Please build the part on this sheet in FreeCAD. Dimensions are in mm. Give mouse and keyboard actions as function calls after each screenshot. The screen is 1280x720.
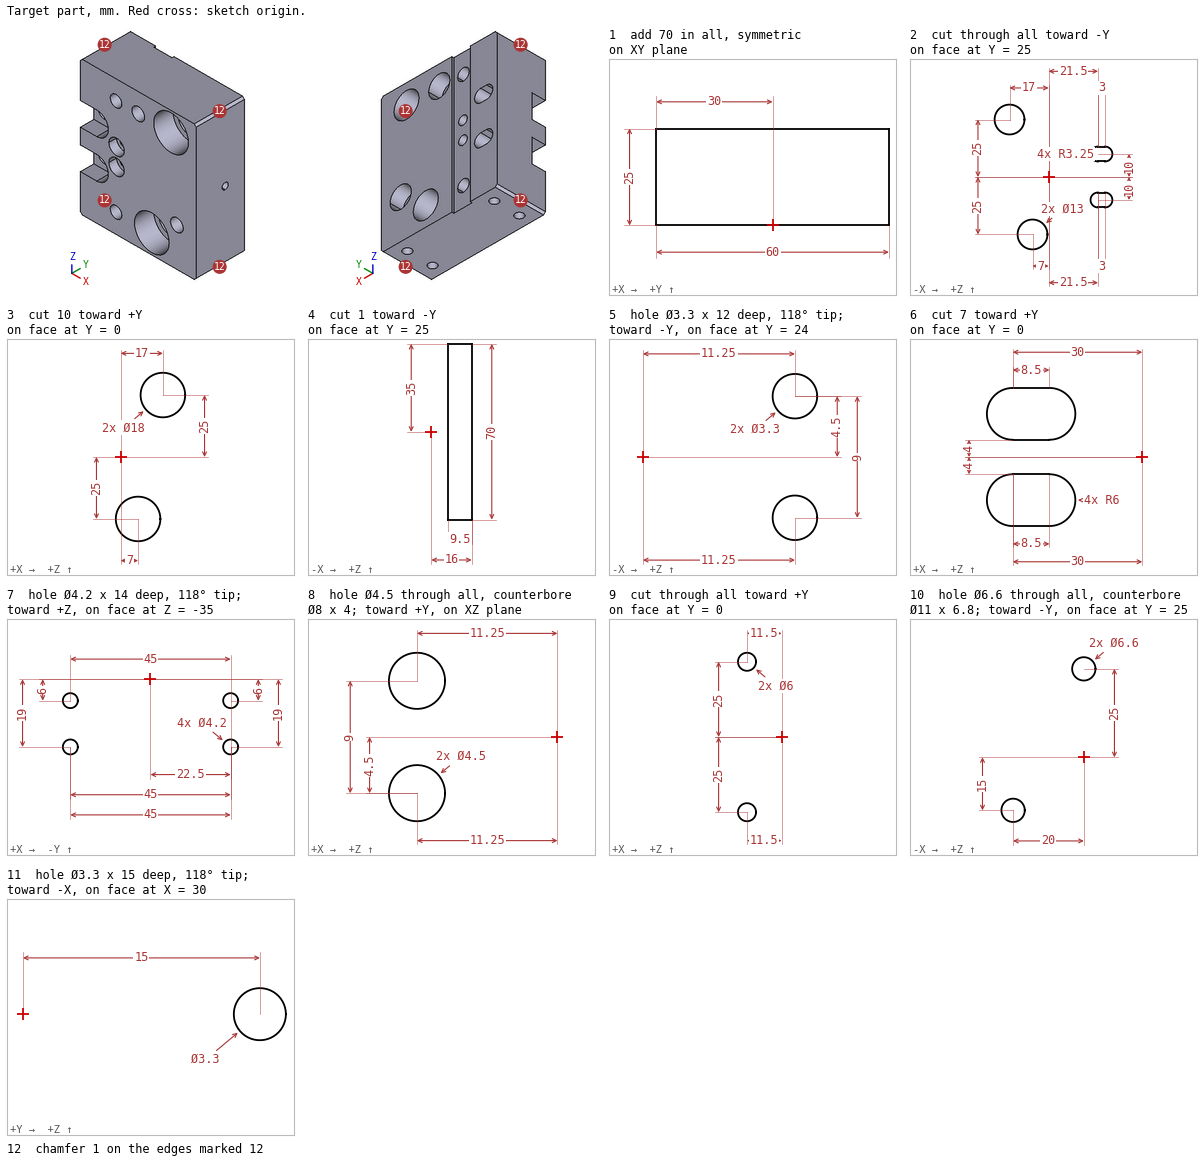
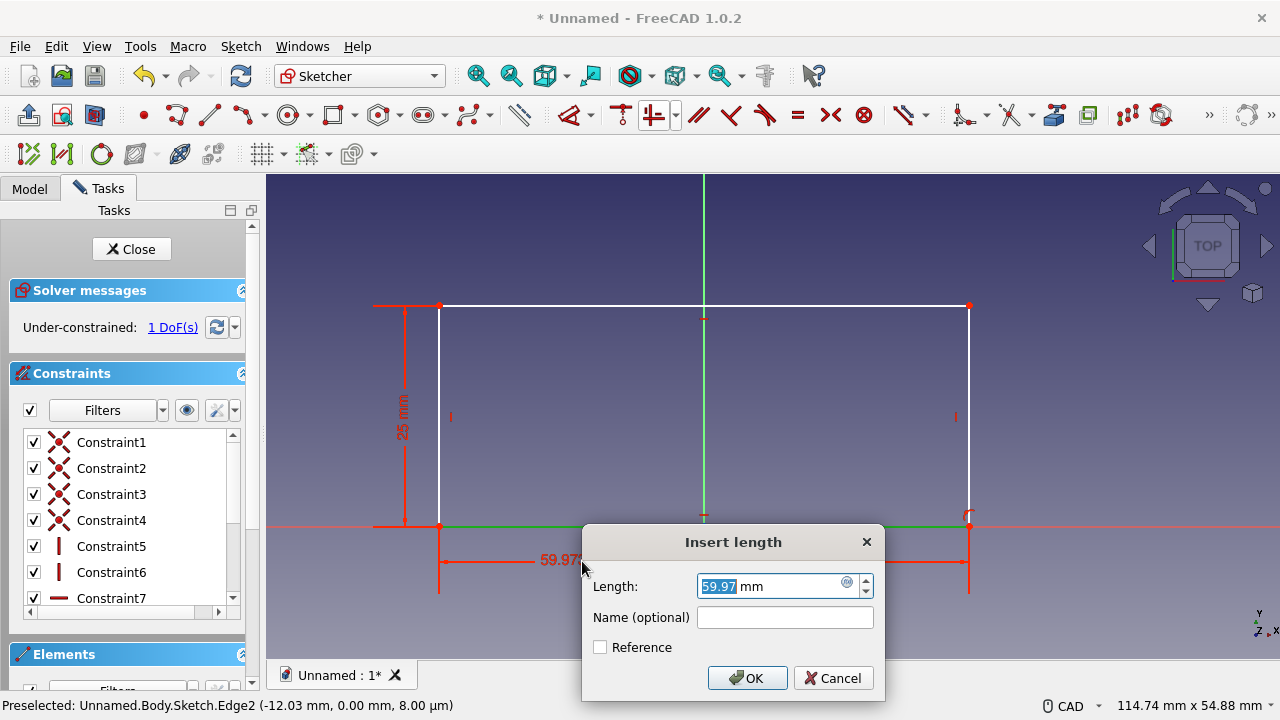
text(60)
key(Return)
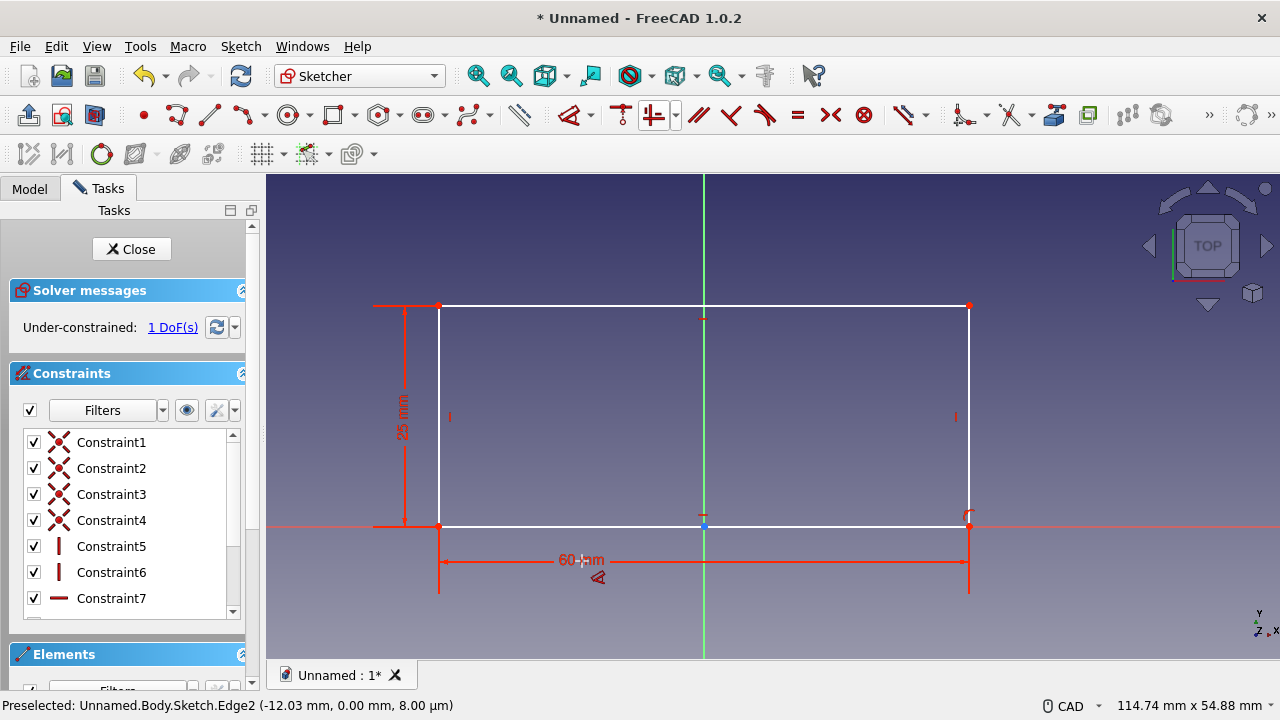
click(439, 306)
click(510, 561)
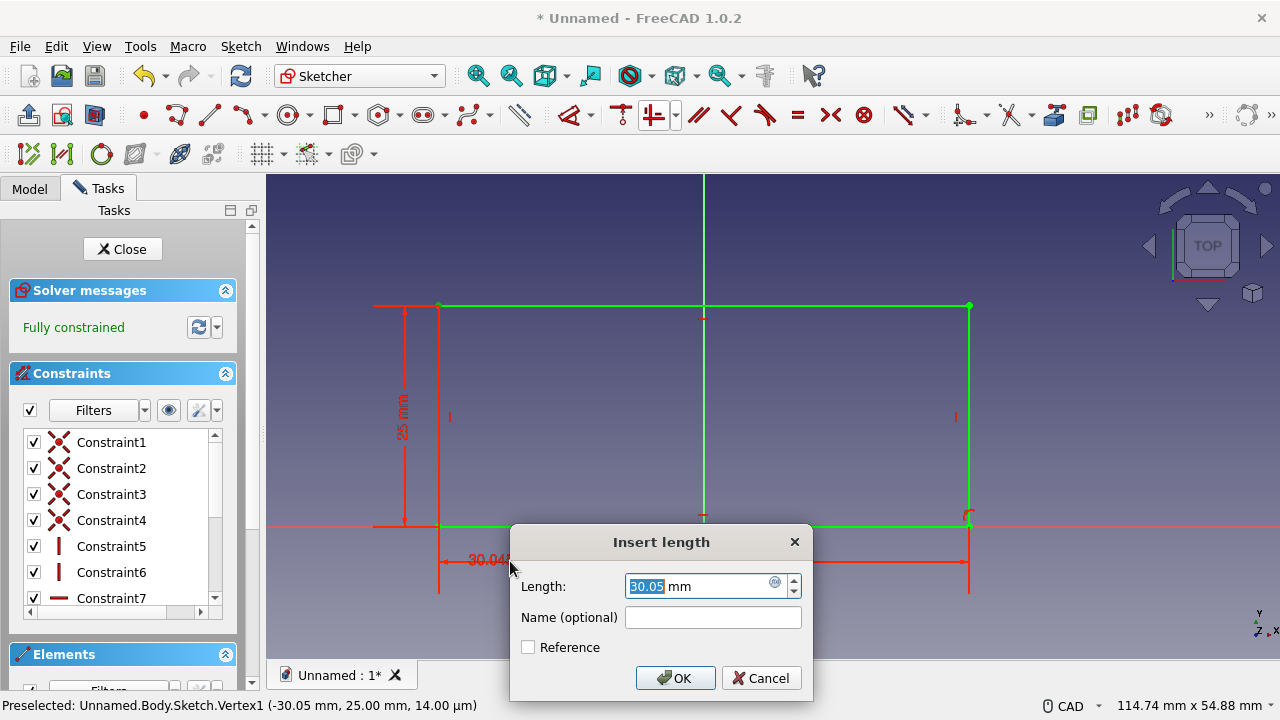
text(30)
key(Return)
key(Escape)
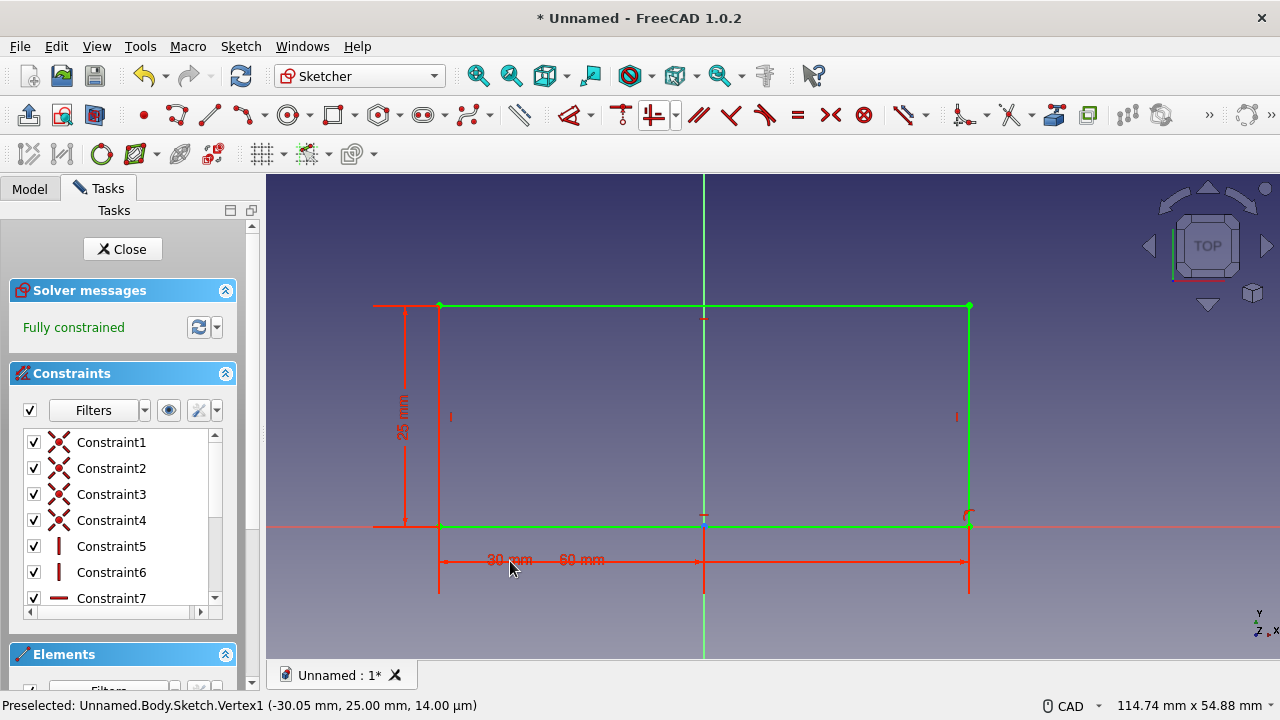
click(123, 249)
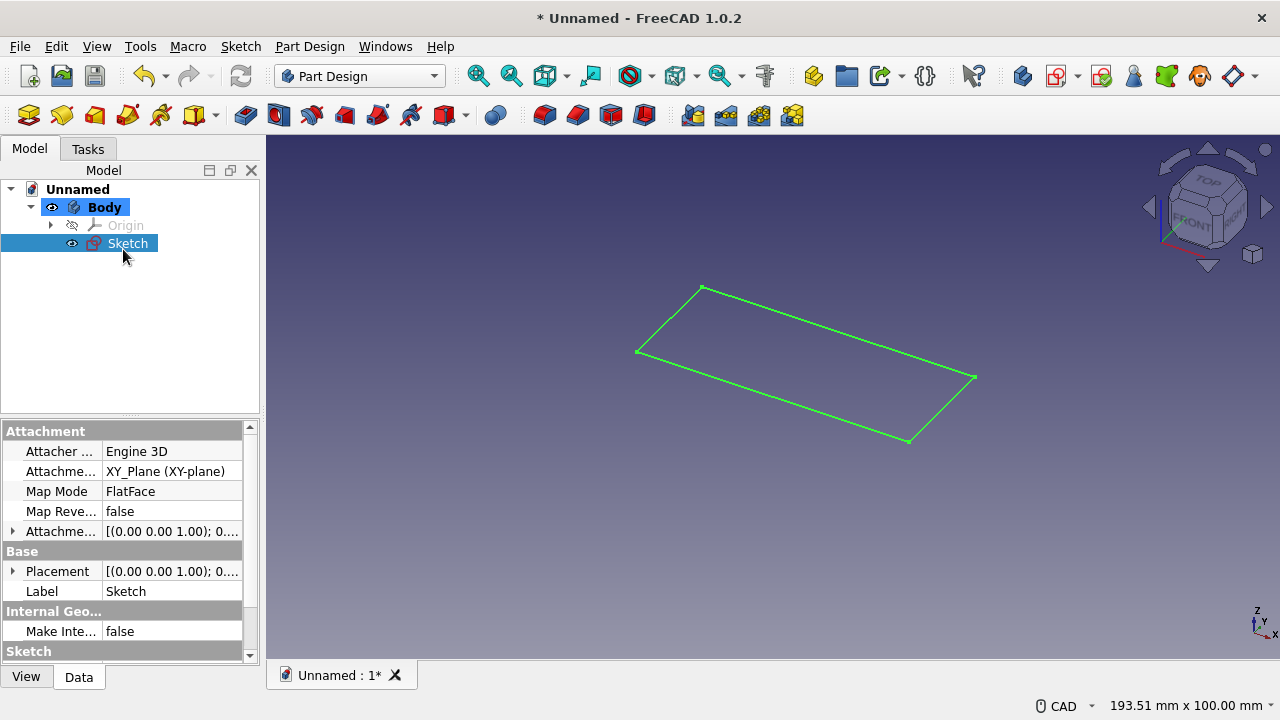
click(29, 116)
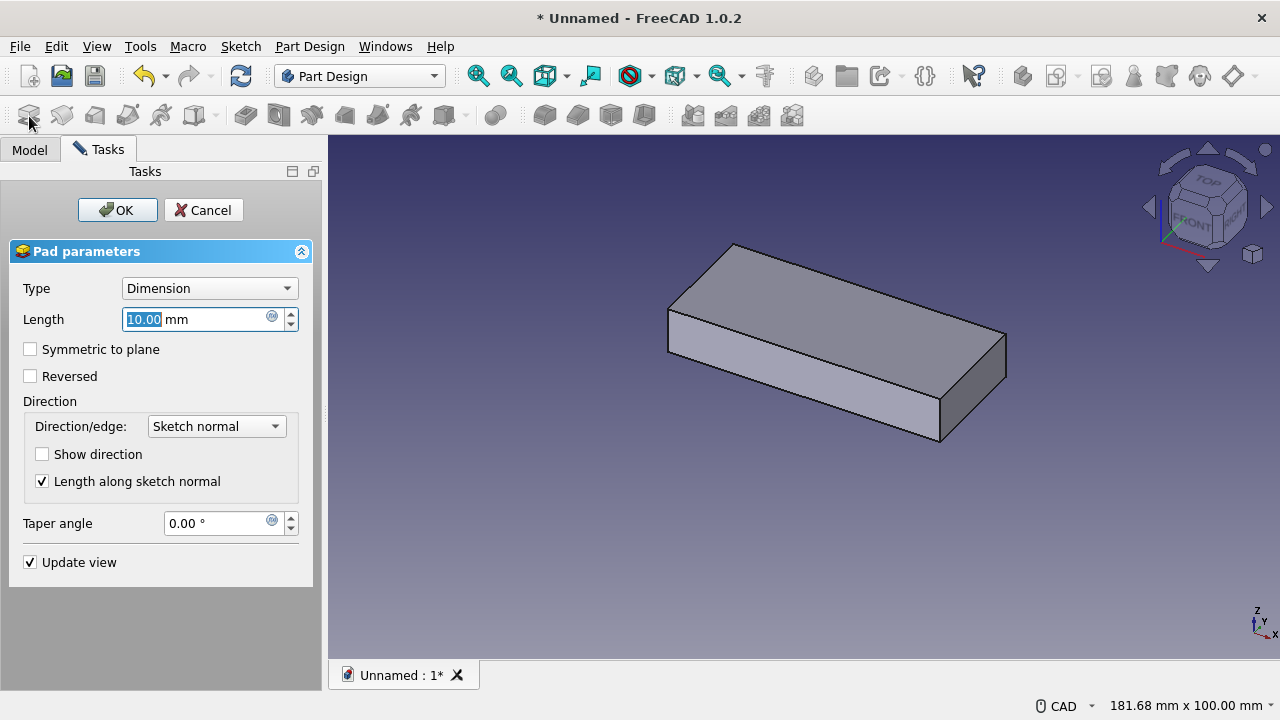
text(70)
key(Tab)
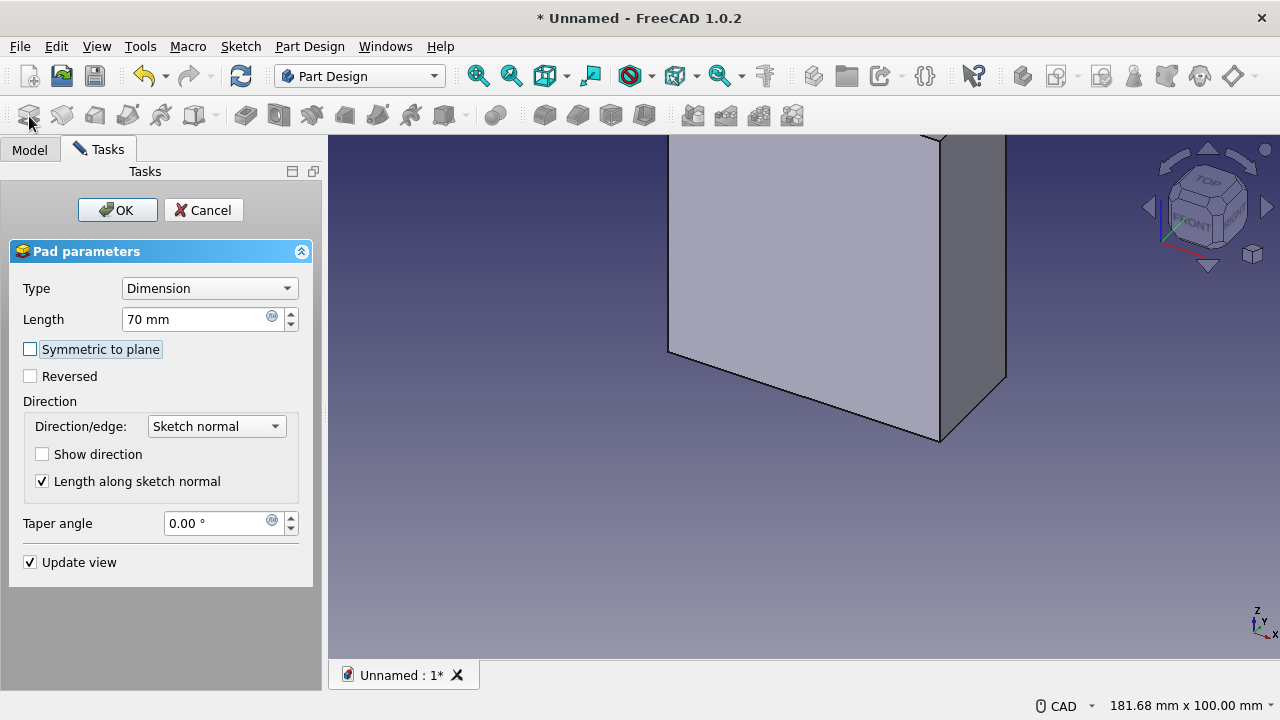
click(31, 349)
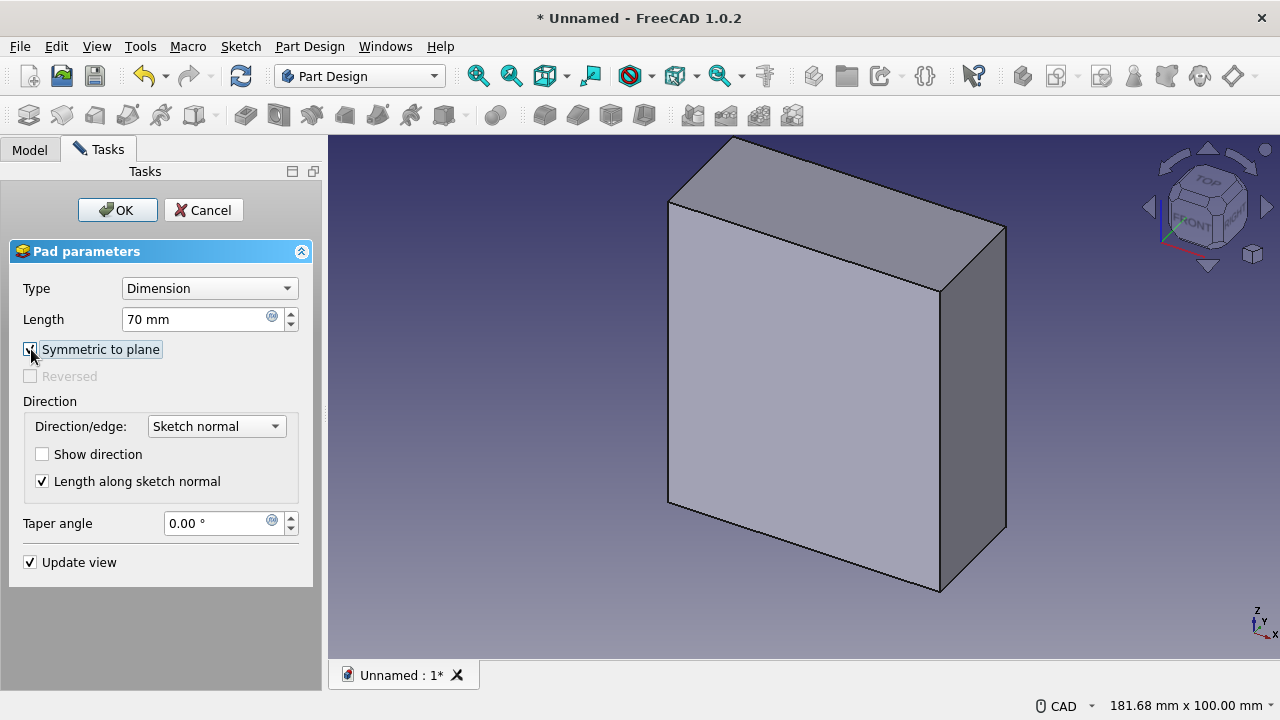
click(118, 210)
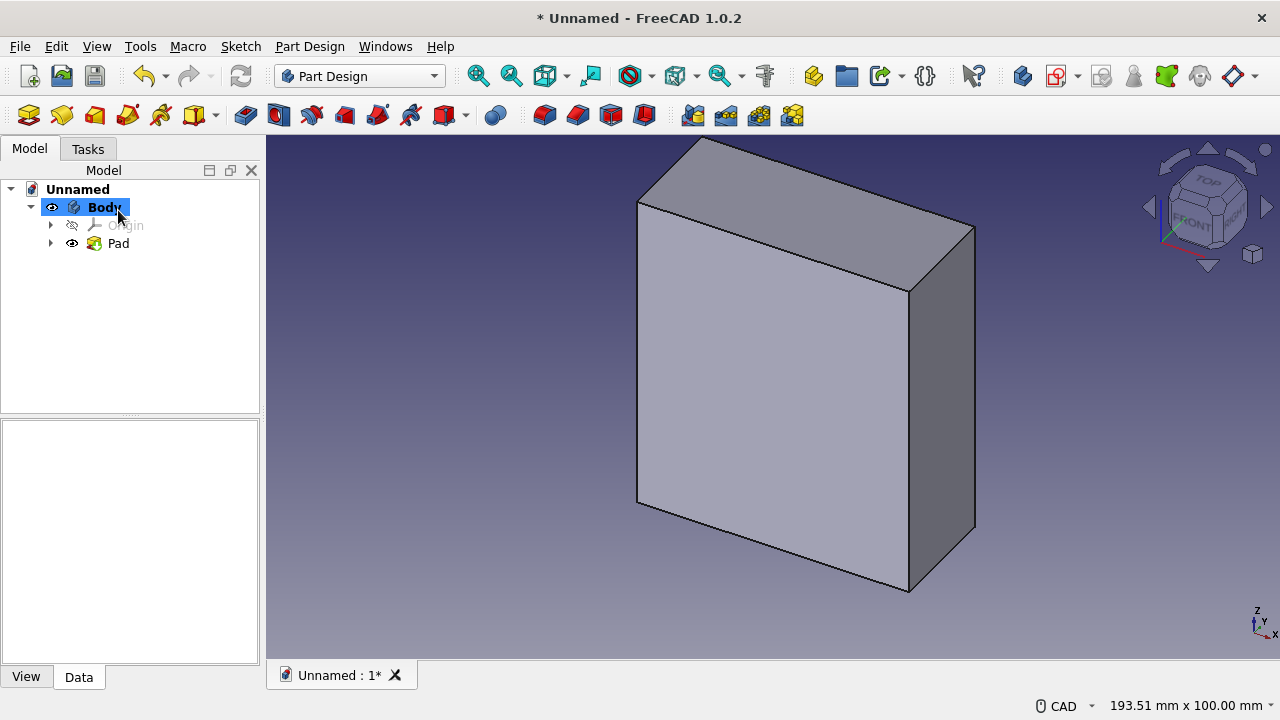
key(4)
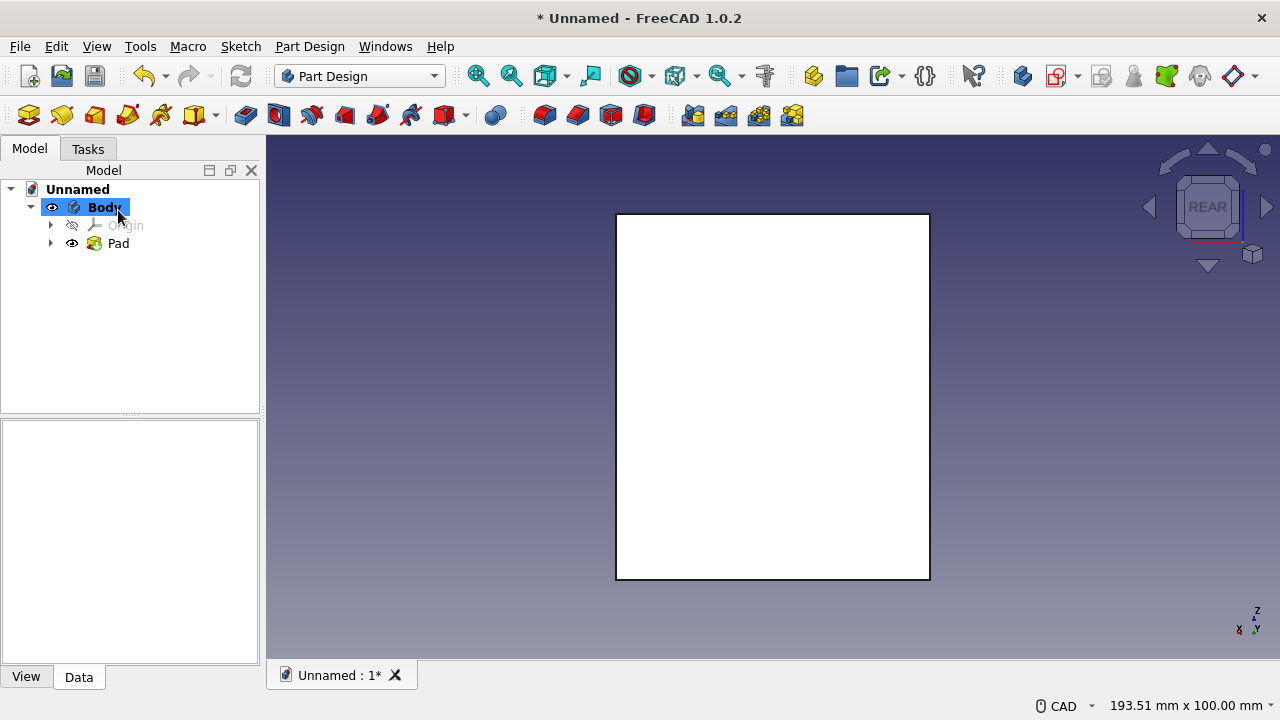
click(773, 396)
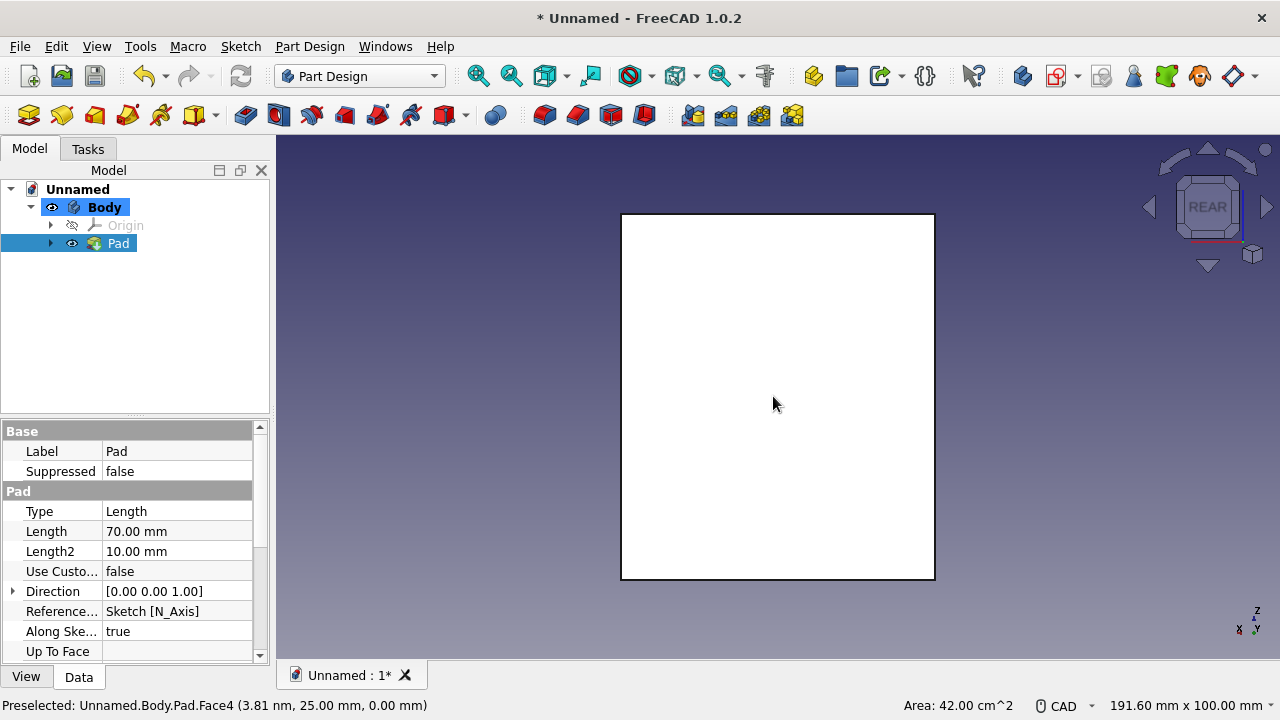
click(1056, 76)